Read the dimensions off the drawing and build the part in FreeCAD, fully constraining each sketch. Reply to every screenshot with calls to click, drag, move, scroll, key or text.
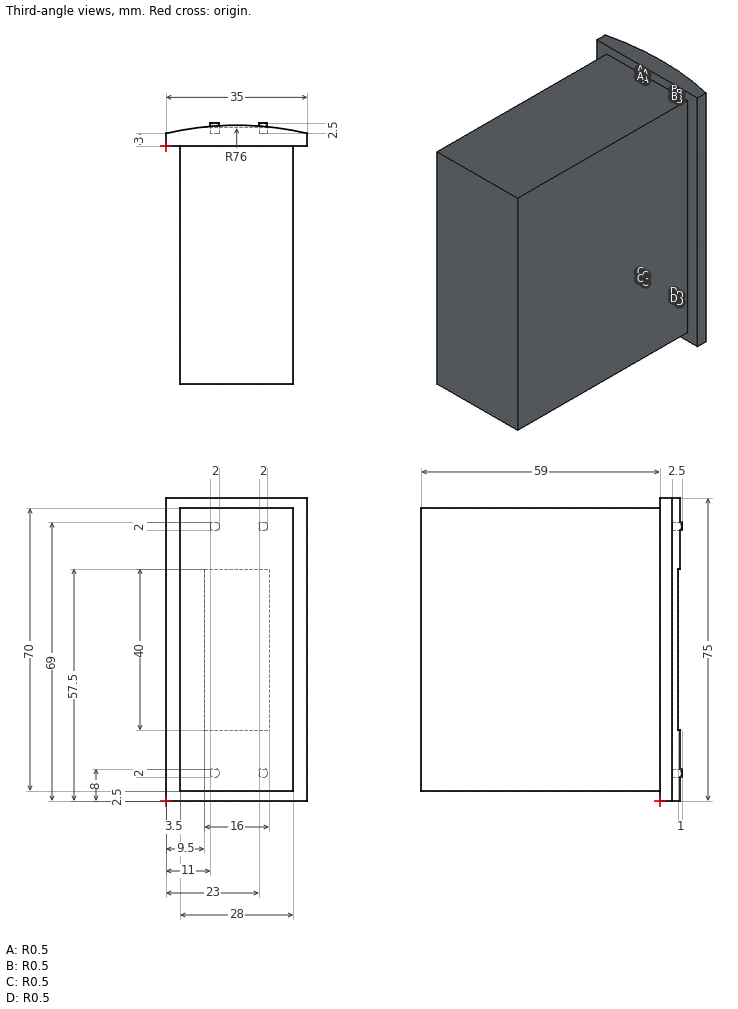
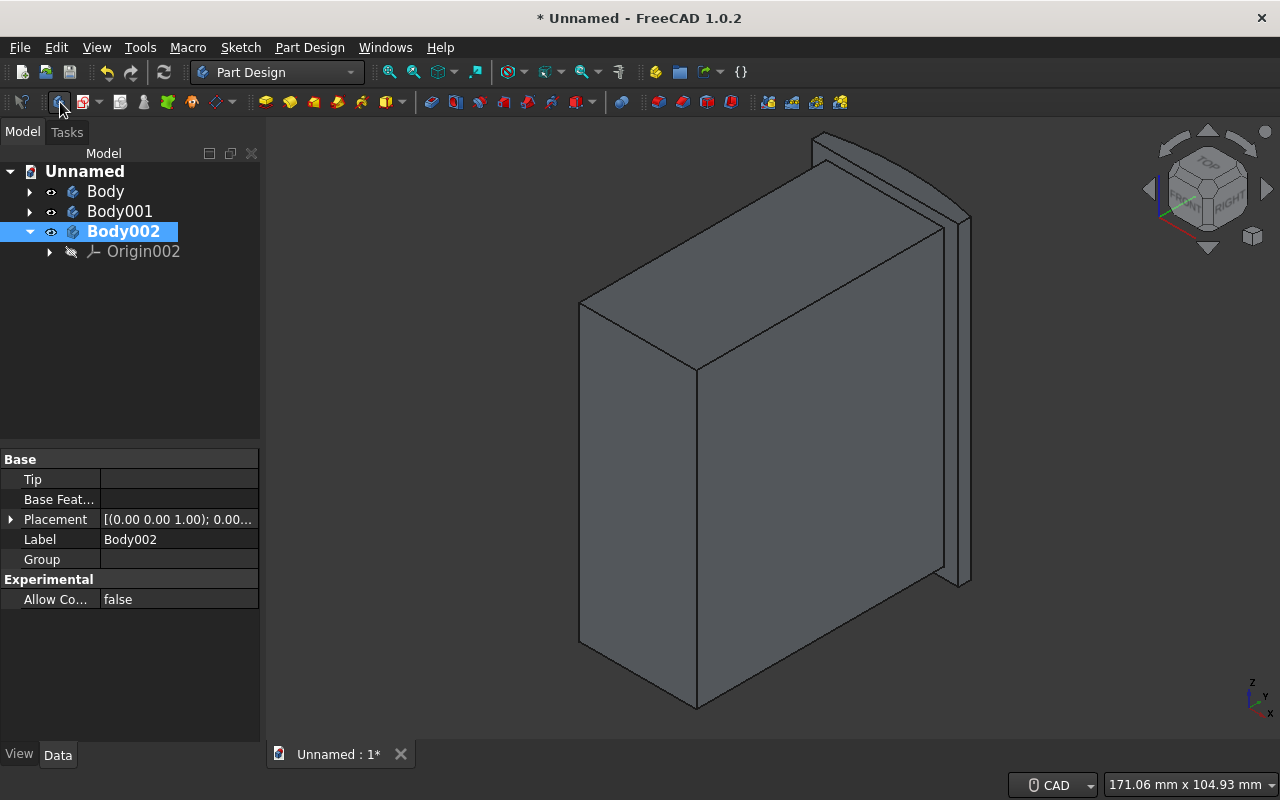
click(50, 252)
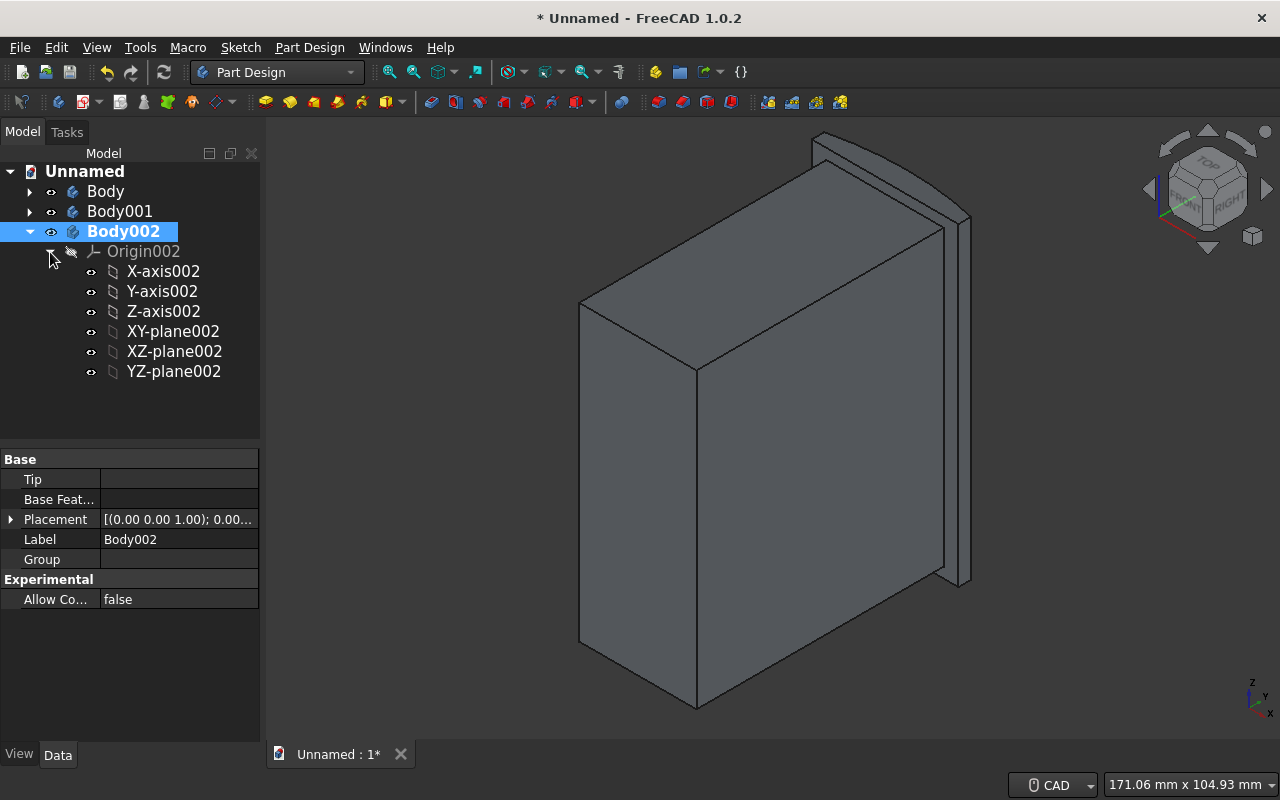
click(136, 352)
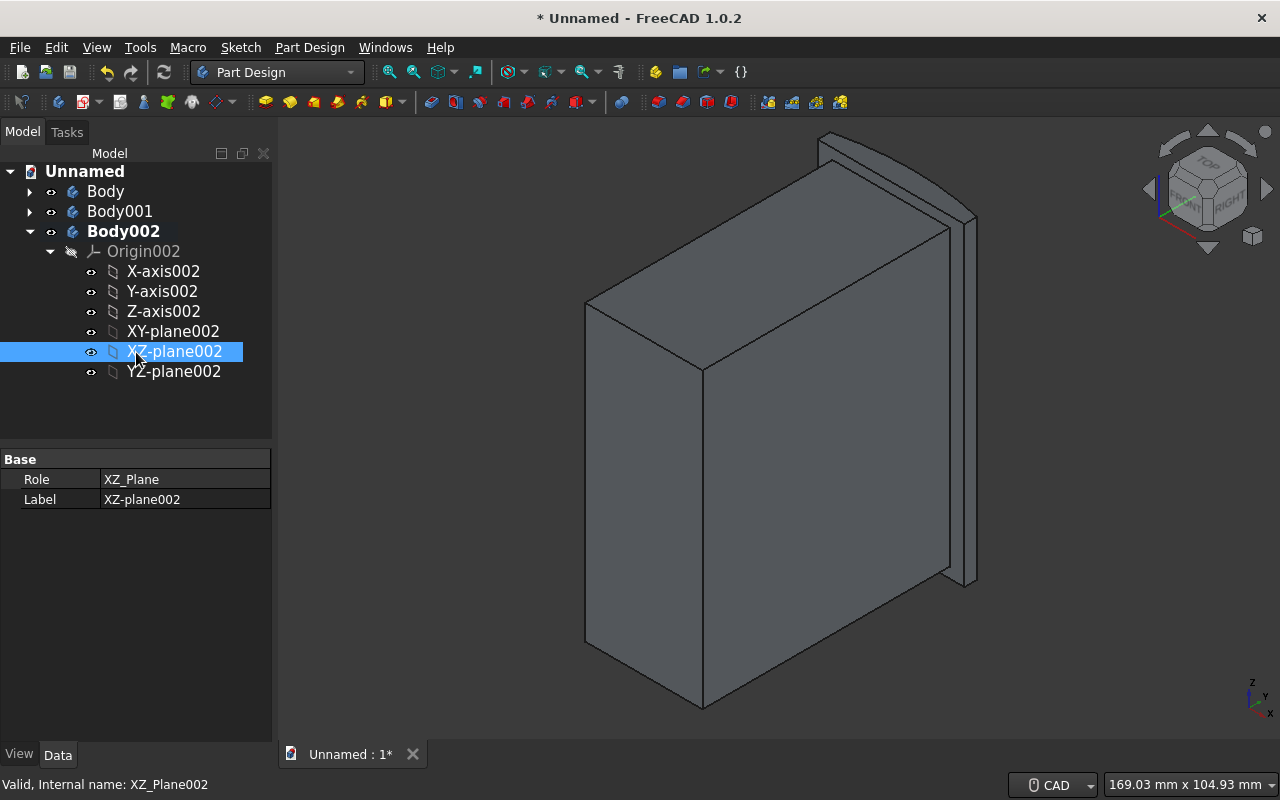
click(216, 102)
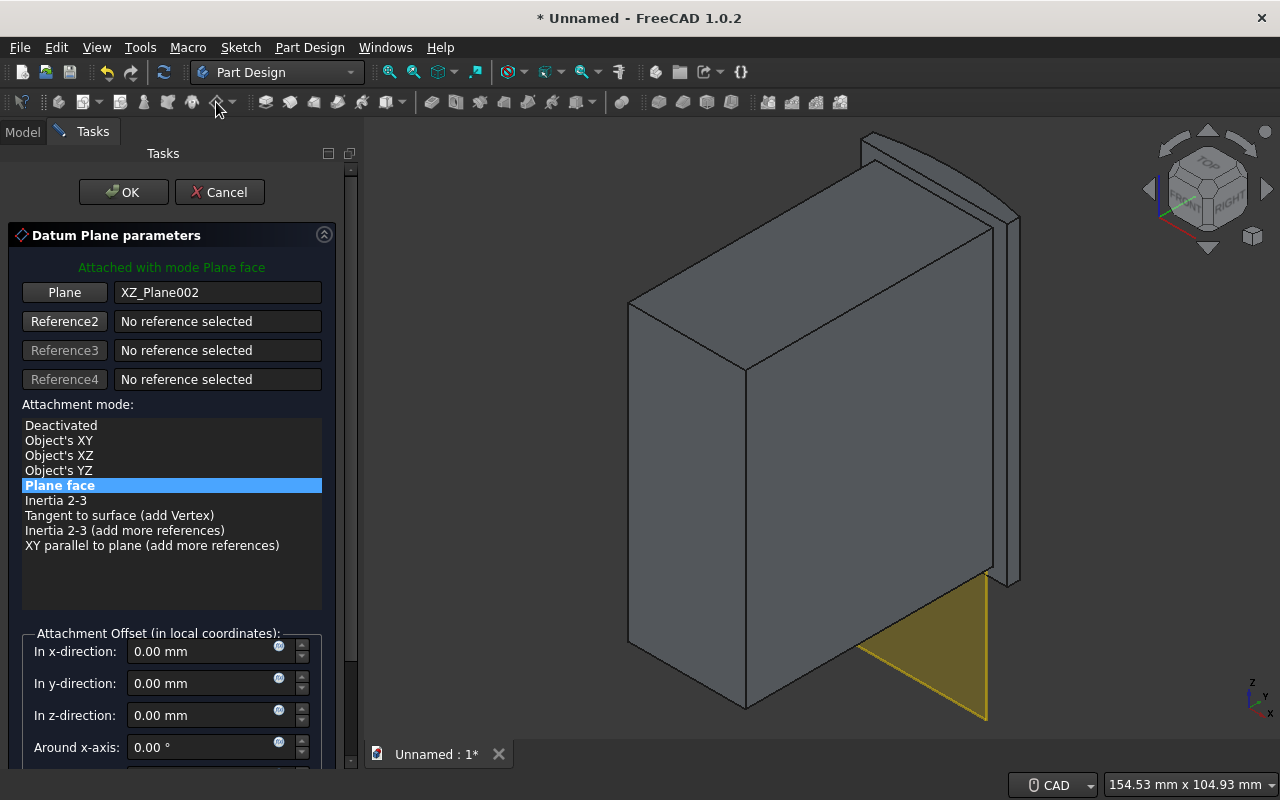
triple_click(210, 715)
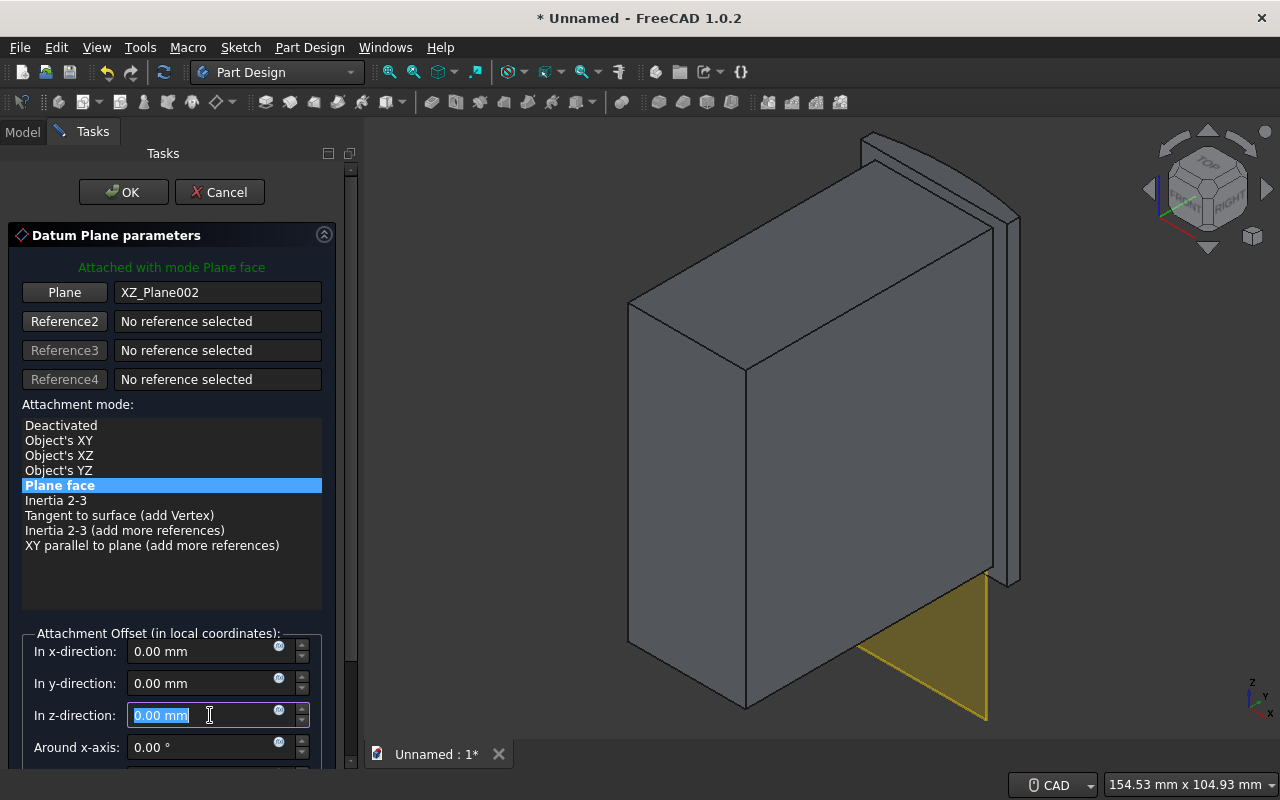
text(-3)
key(Tab)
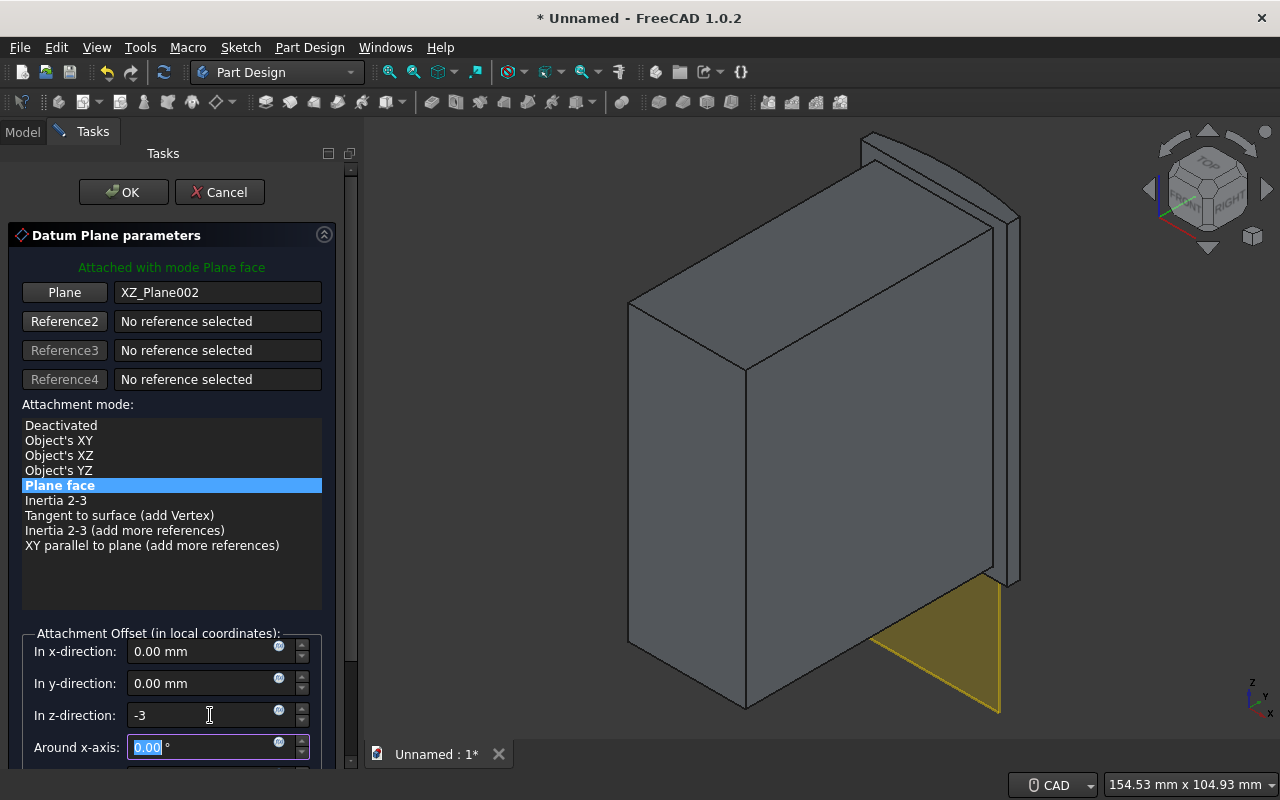
click(124, 192)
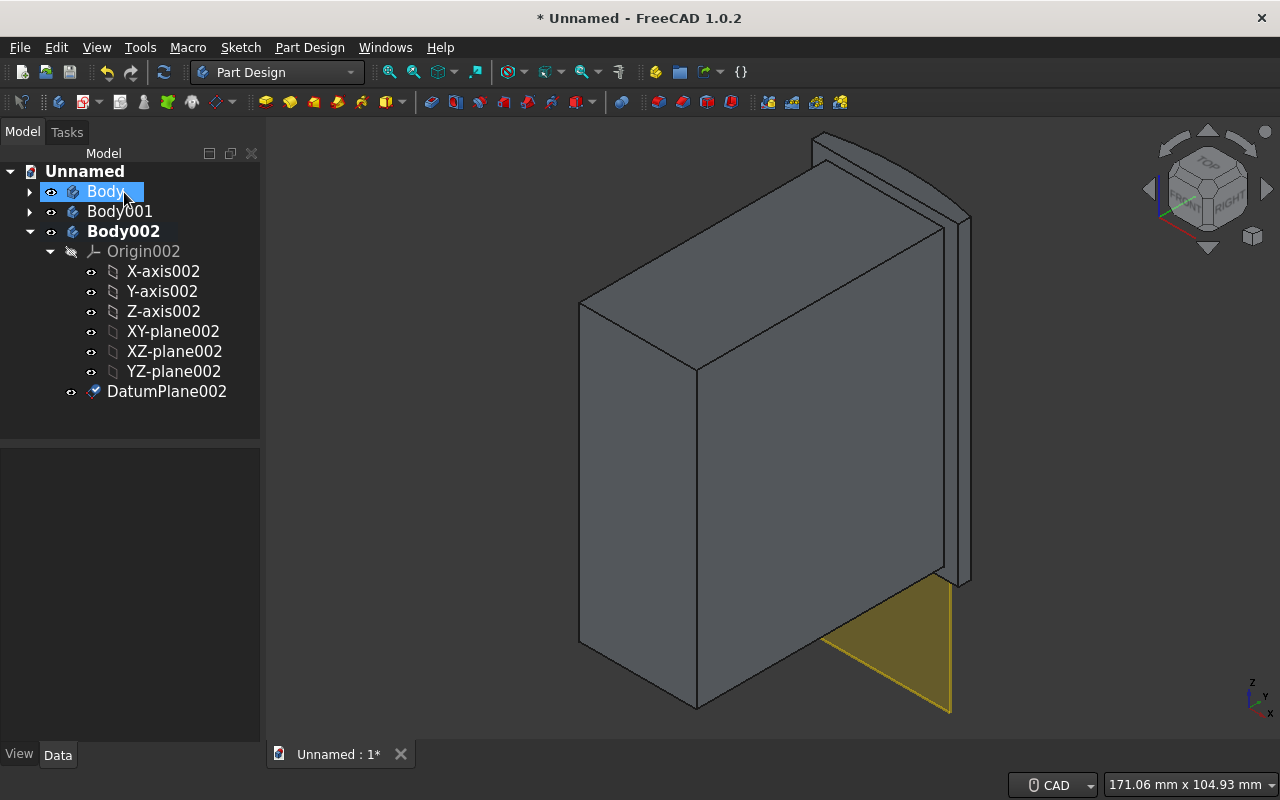
click(116, 392)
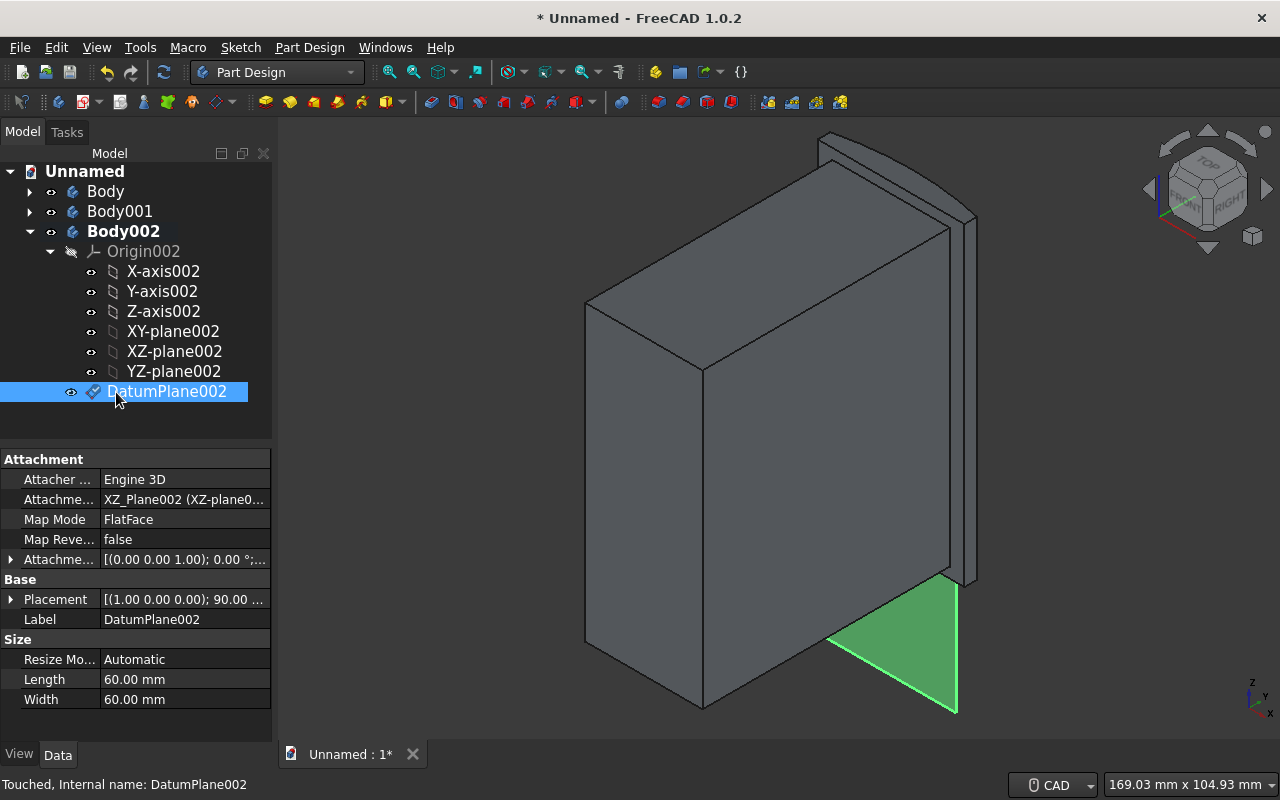
click(84, 102)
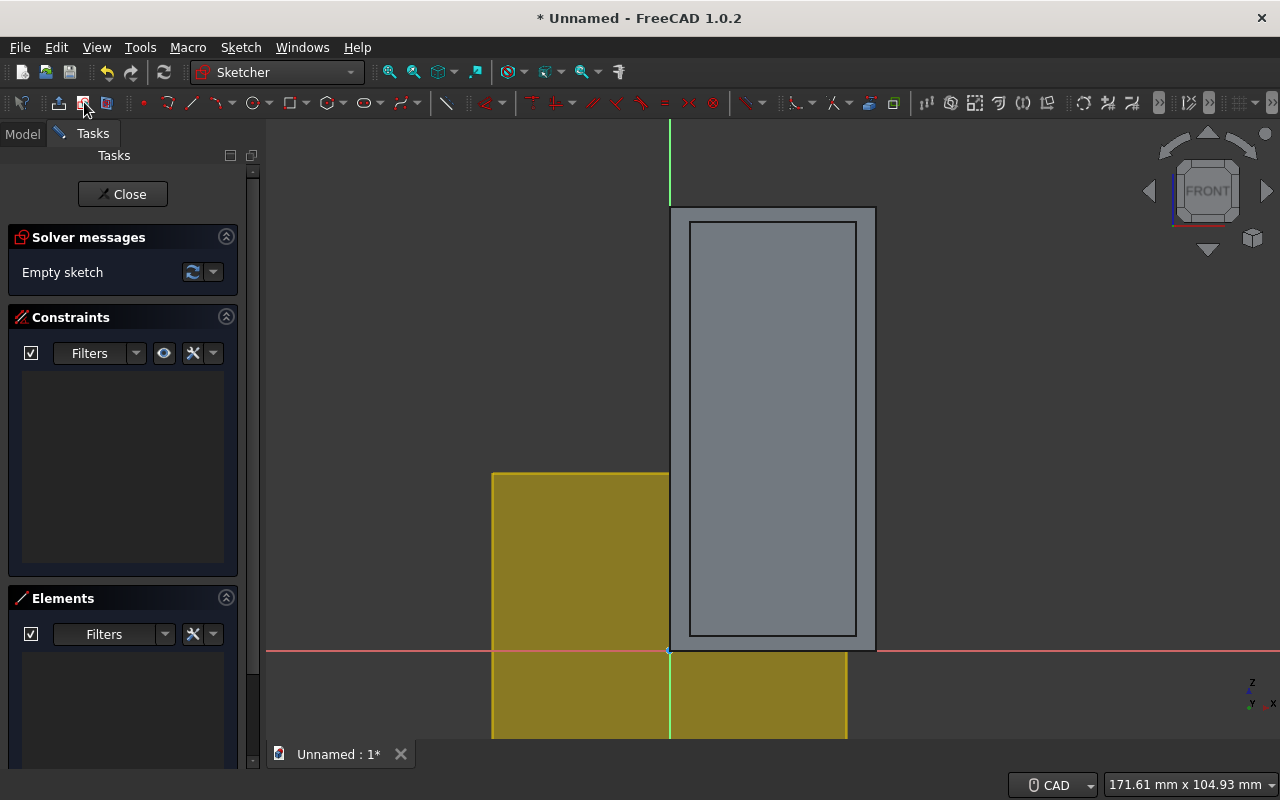
scroll(817, 239, up, 15)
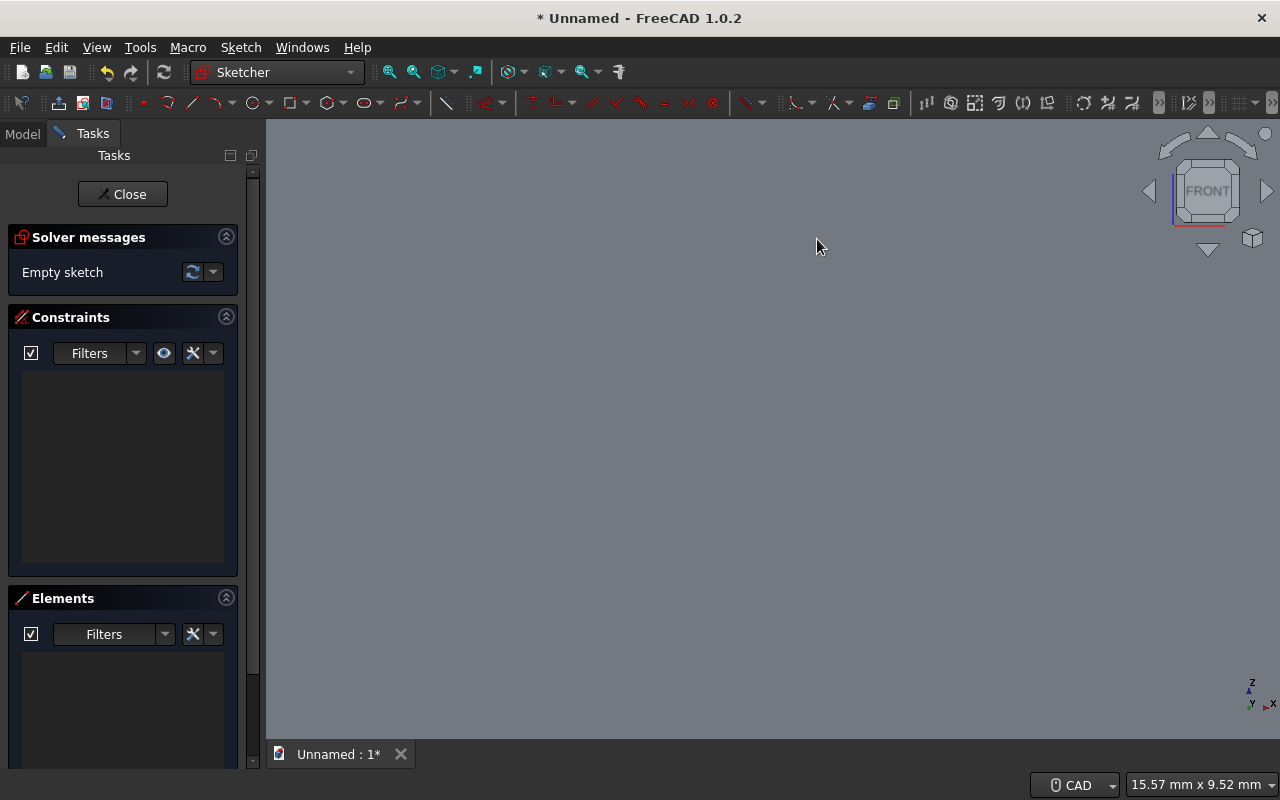
scroll(682, 435, up, 3)